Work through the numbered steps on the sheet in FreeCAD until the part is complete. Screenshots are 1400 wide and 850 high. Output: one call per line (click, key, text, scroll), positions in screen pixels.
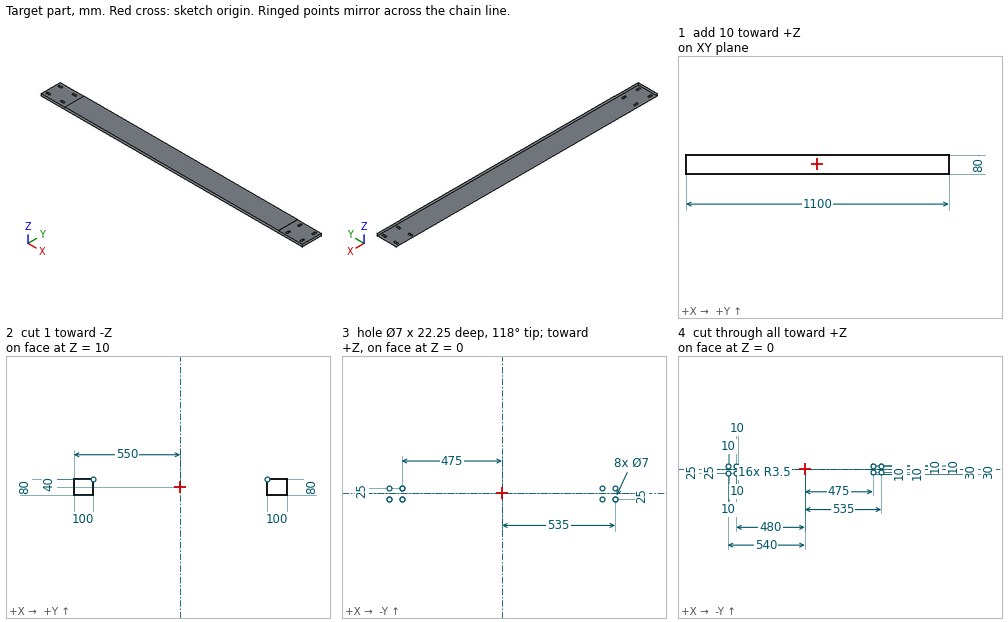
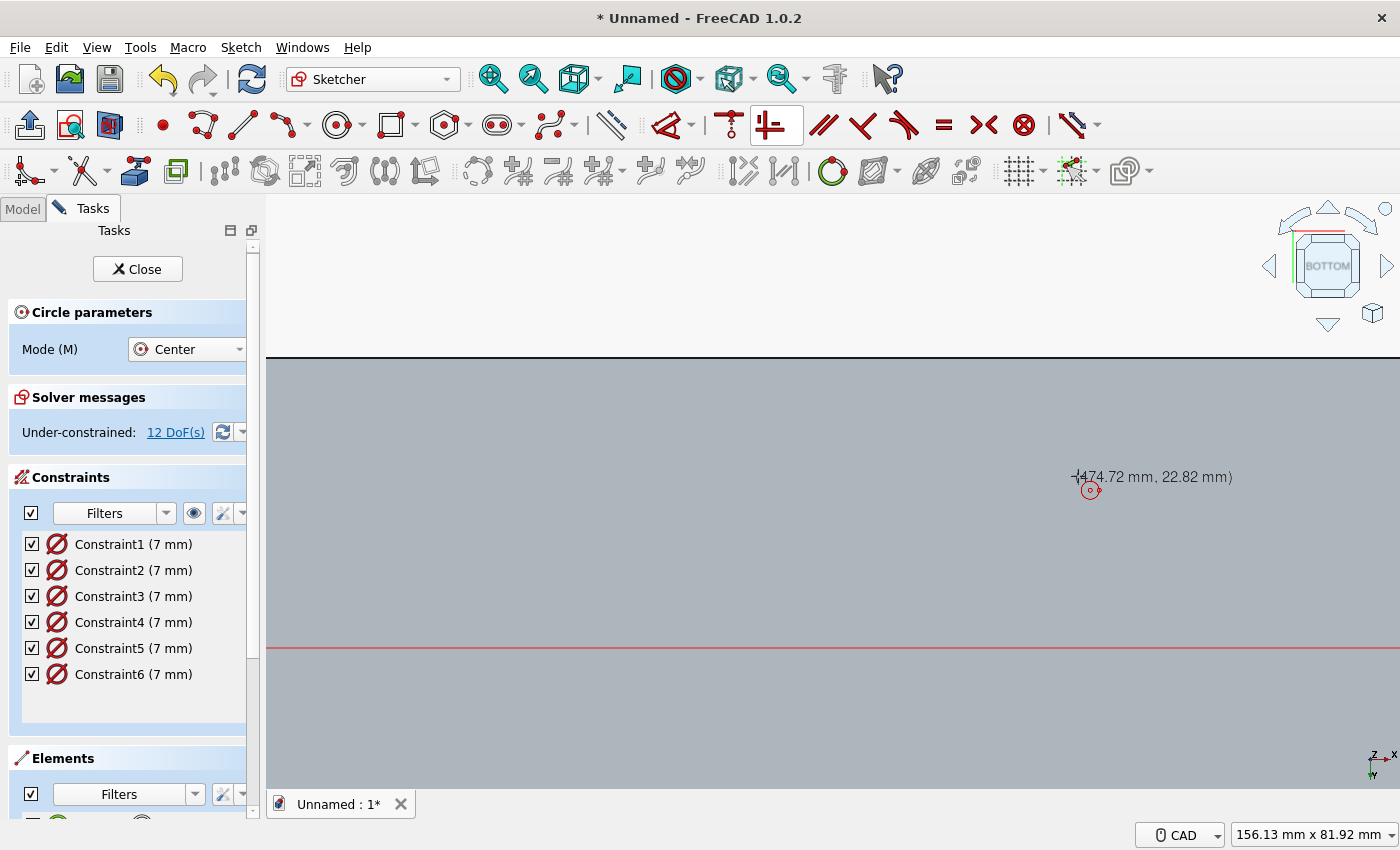
scroll(1078, 476, down, 12)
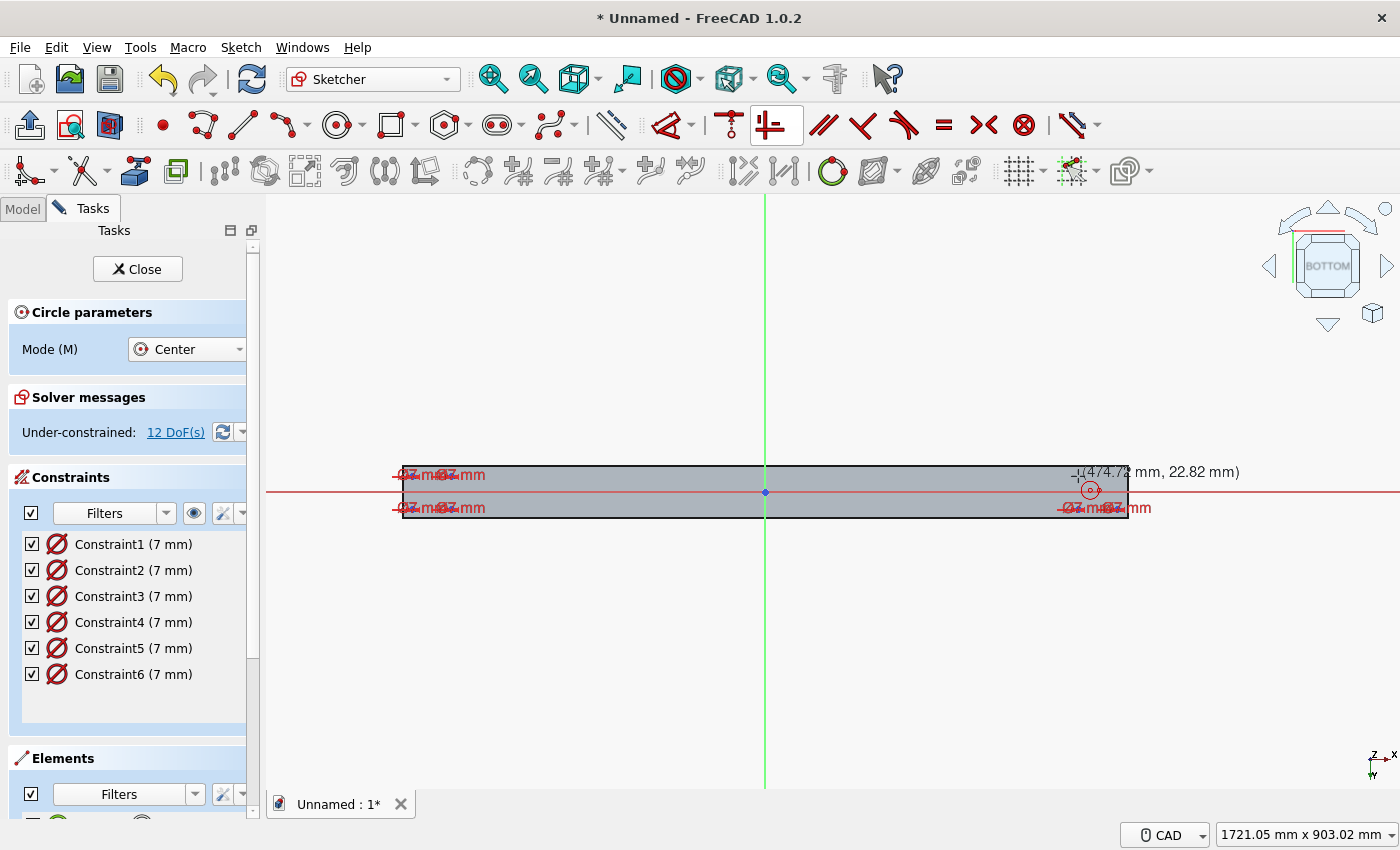
click(1078, 476)
move(1080, 474)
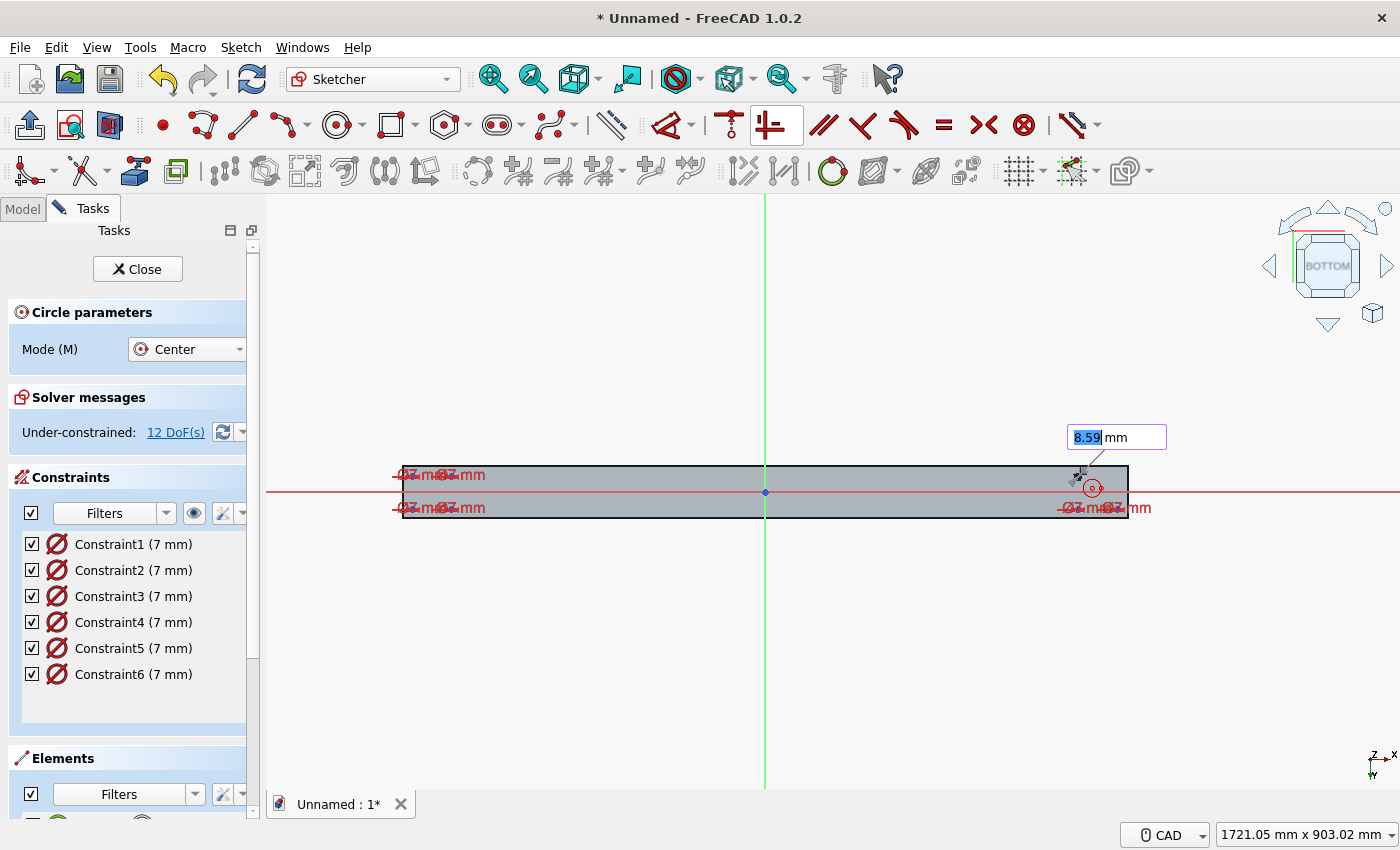
text(7)
key(Return)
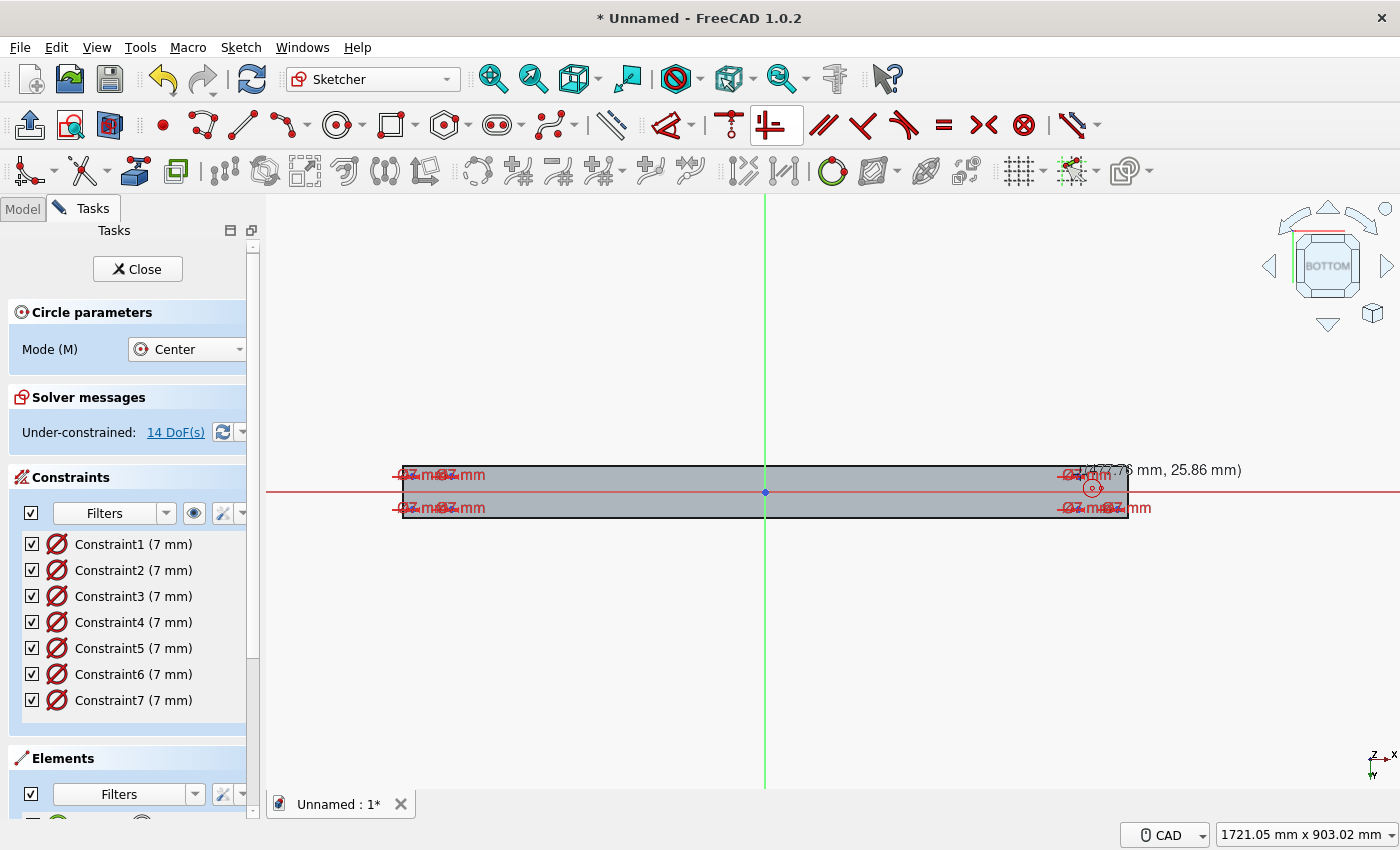
scroll(1118, 476, up, 12)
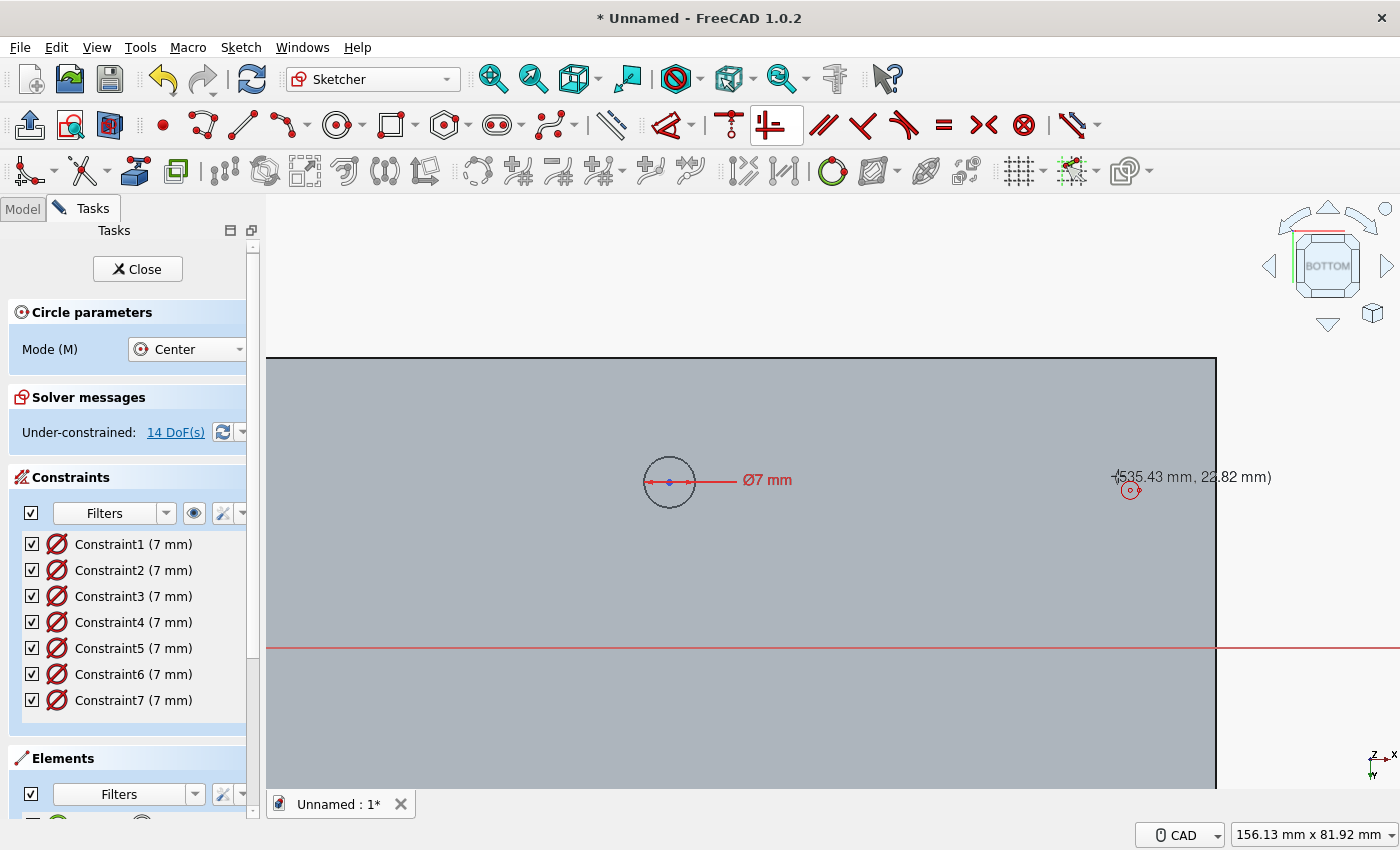
scroll(1118, 476, down, 12)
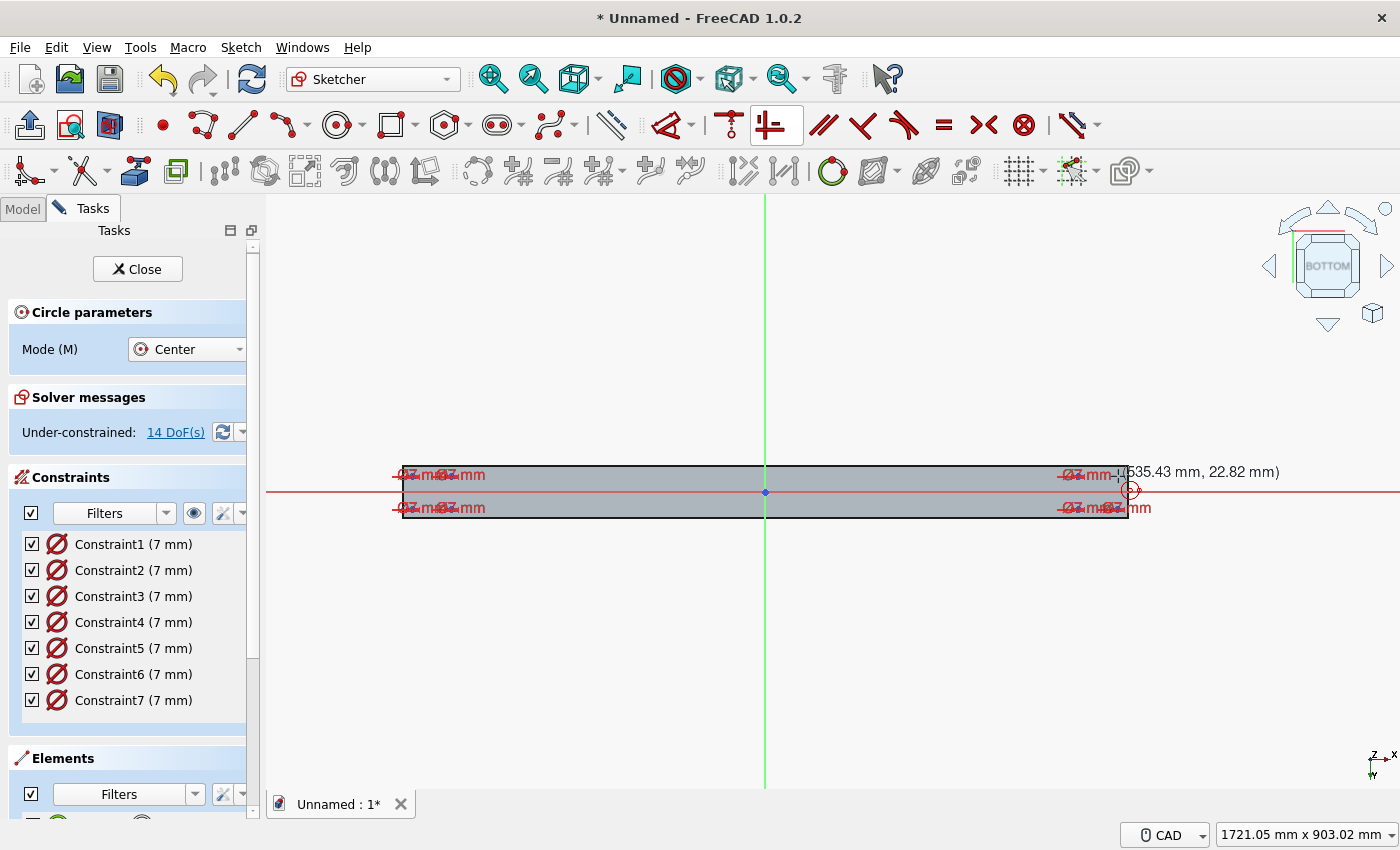
click(1118, 476)
move(1119, 474)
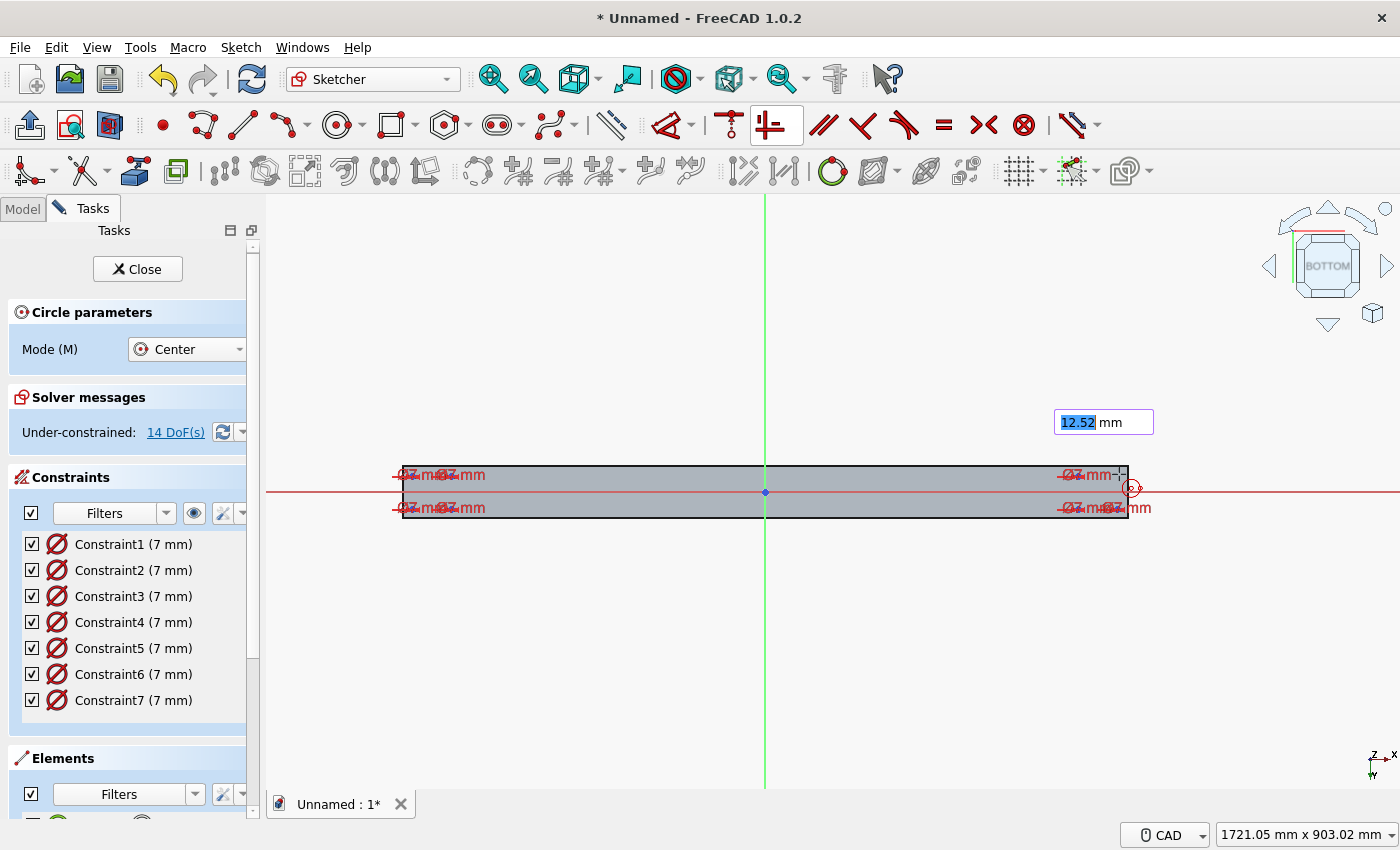
text(7)
key(Return)
key(Escape)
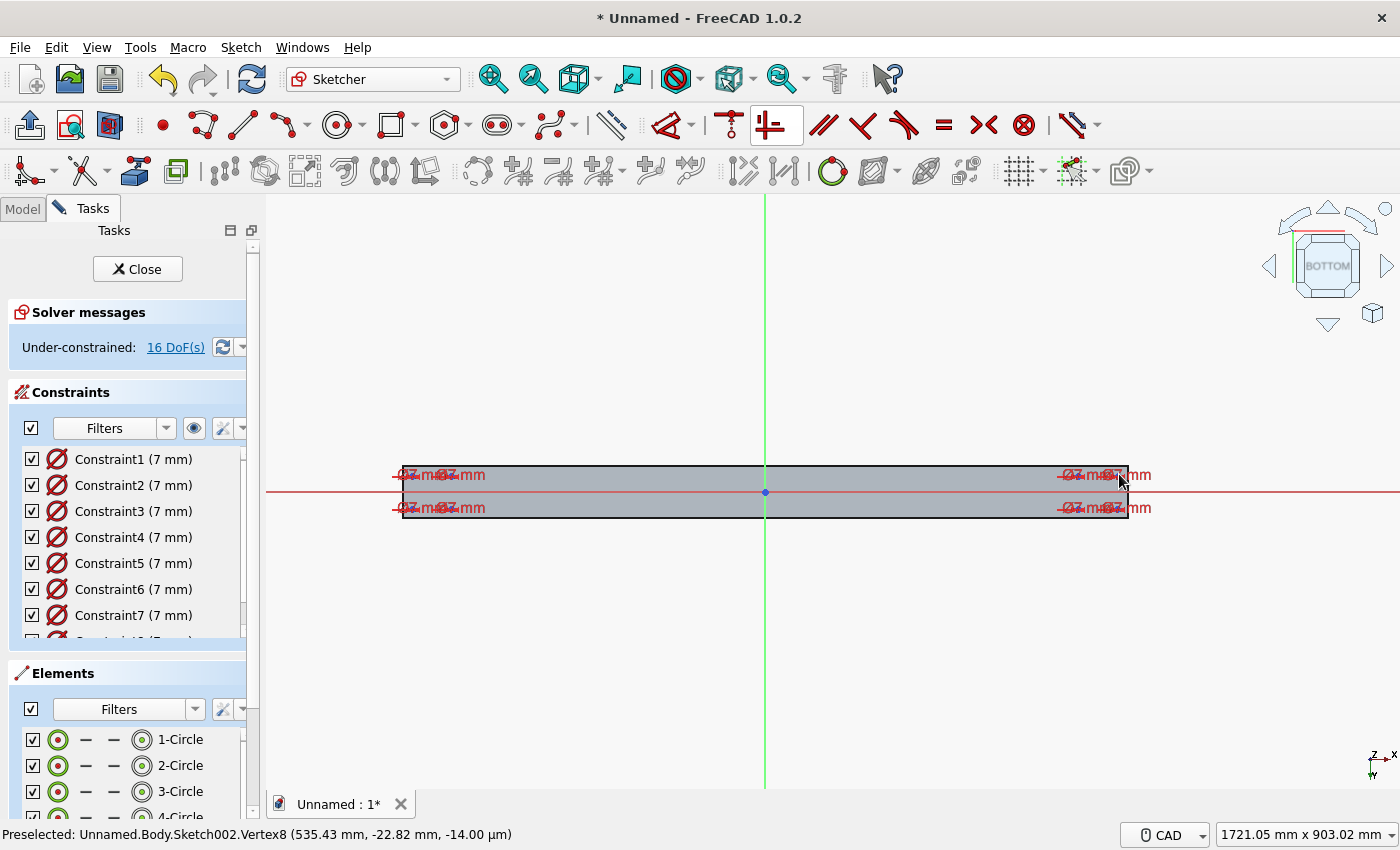
click(1118, 510)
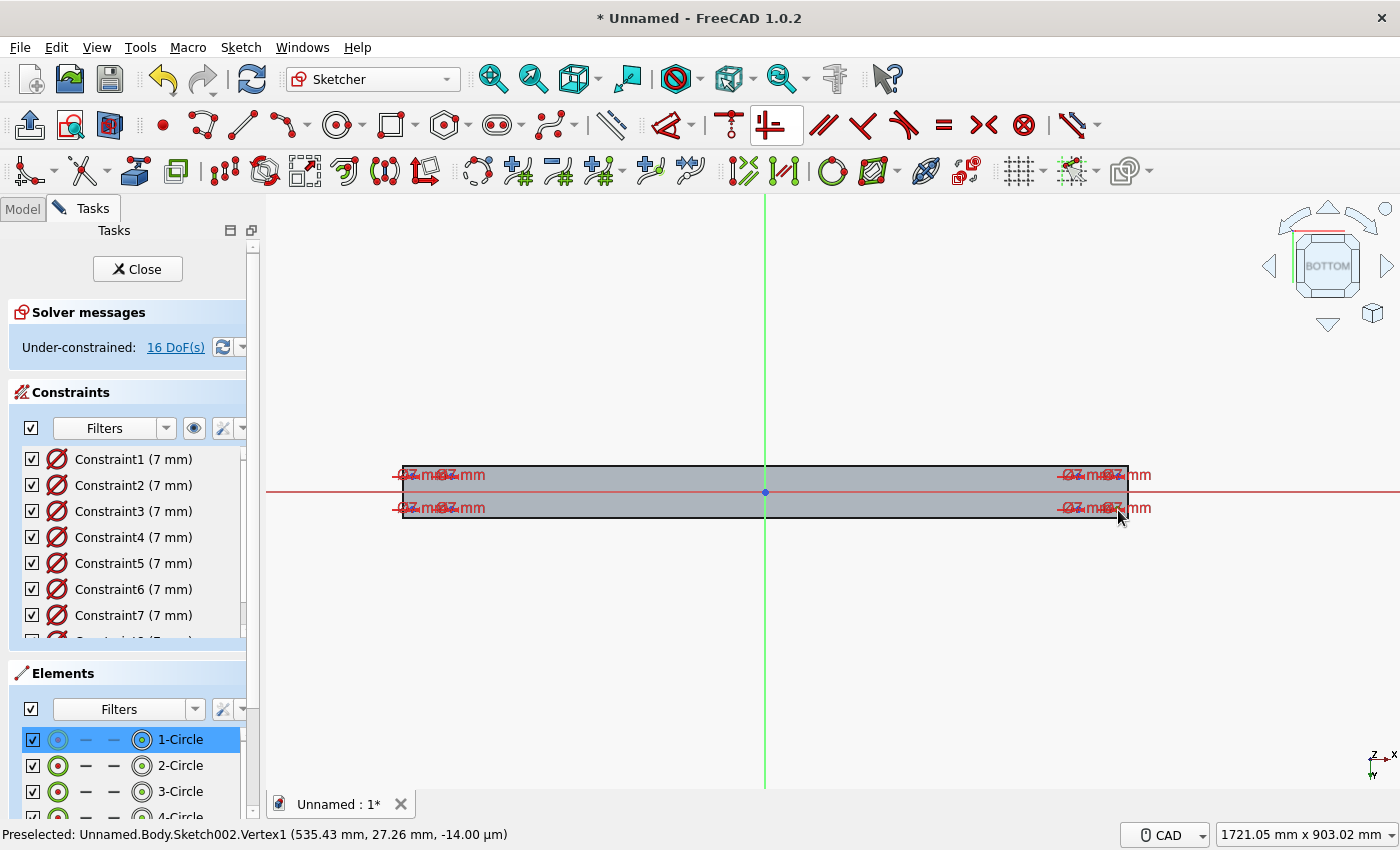
click(413, 510)